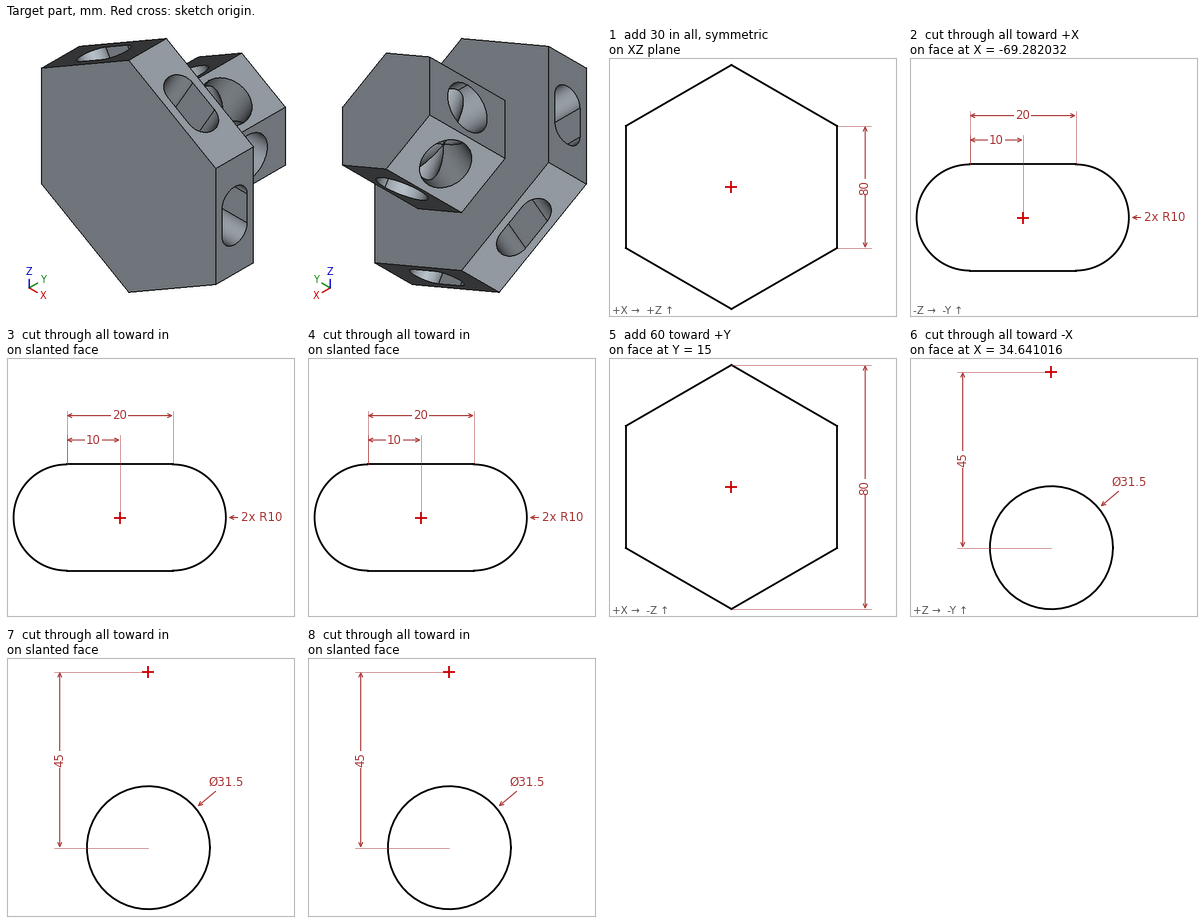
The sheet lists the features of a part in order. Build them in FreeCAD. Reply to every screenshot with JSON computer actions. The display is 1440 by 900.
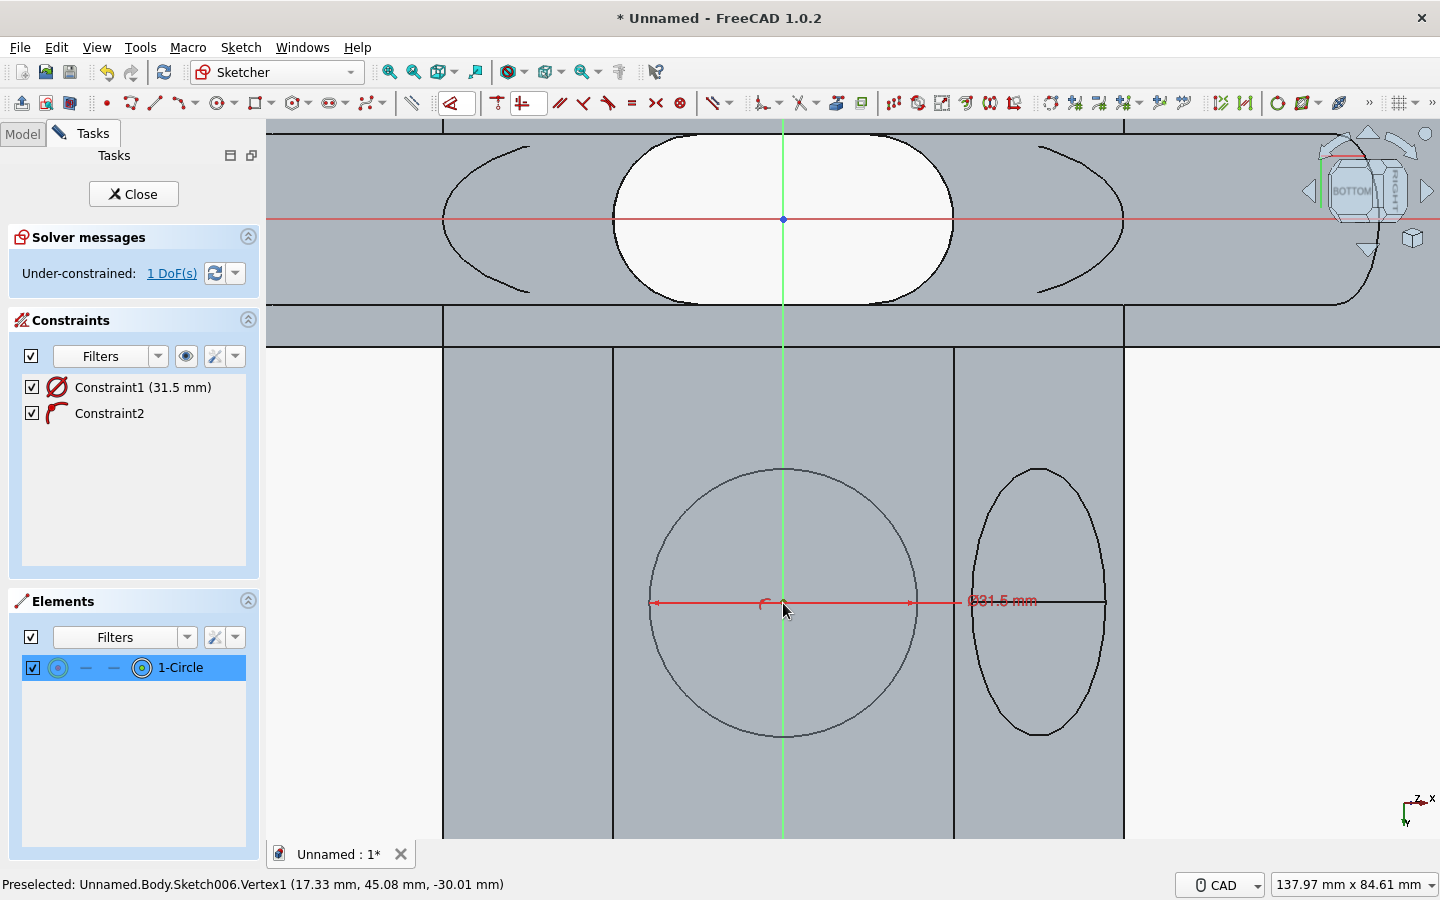
{"action": "left_click", "coordinate": [470, 104]}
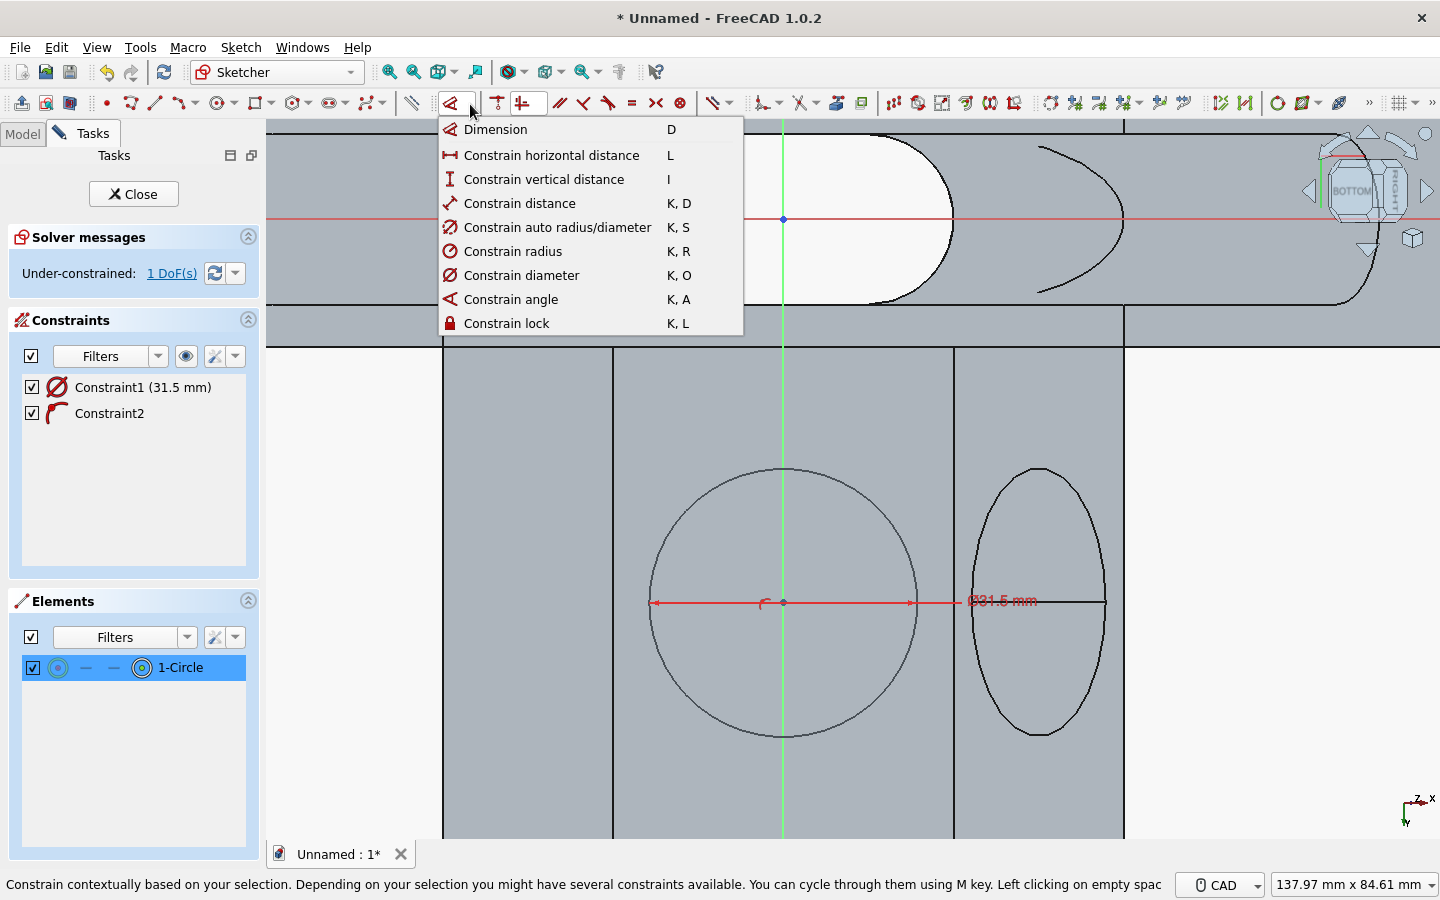
{"action": "left_click", "coordinate": [591, 179]}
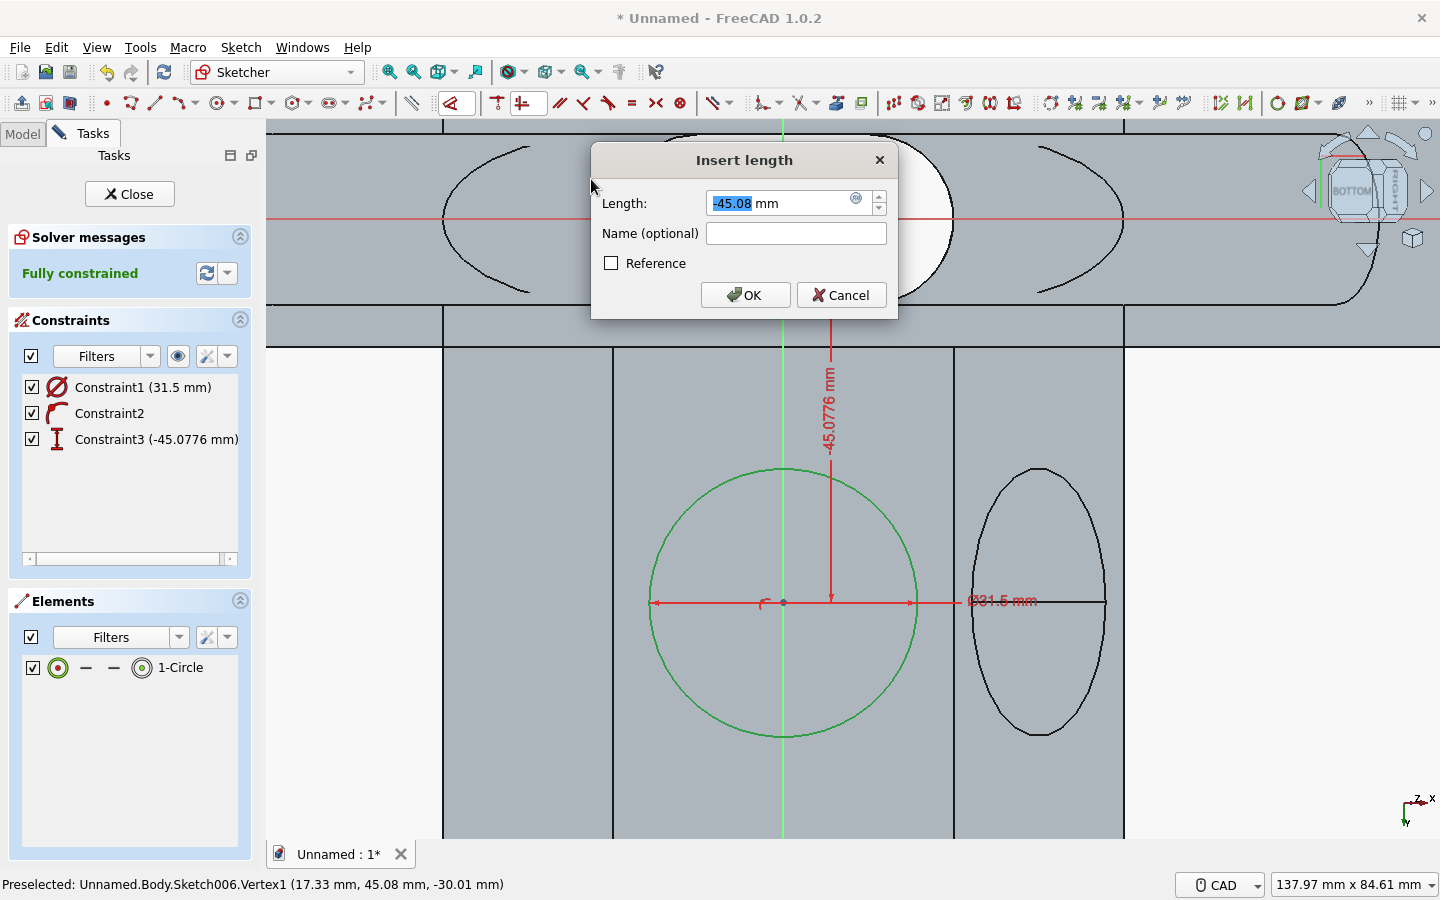
{"action": "type", "text": "-45"}
{"action": "key", "text": "Return"}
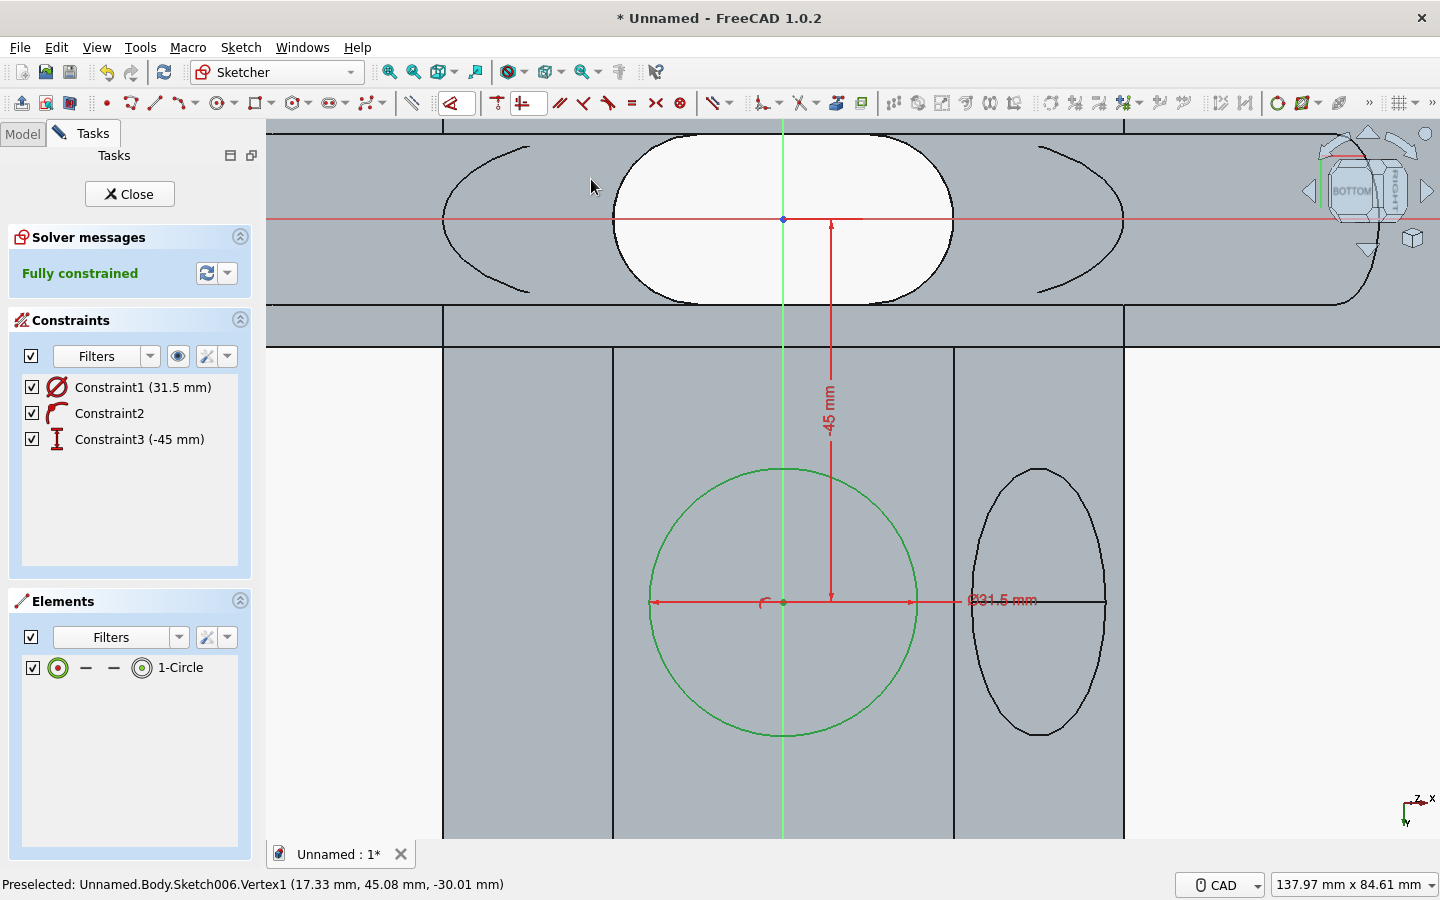
{"action": "left_click", "coordinate": [130, 194]}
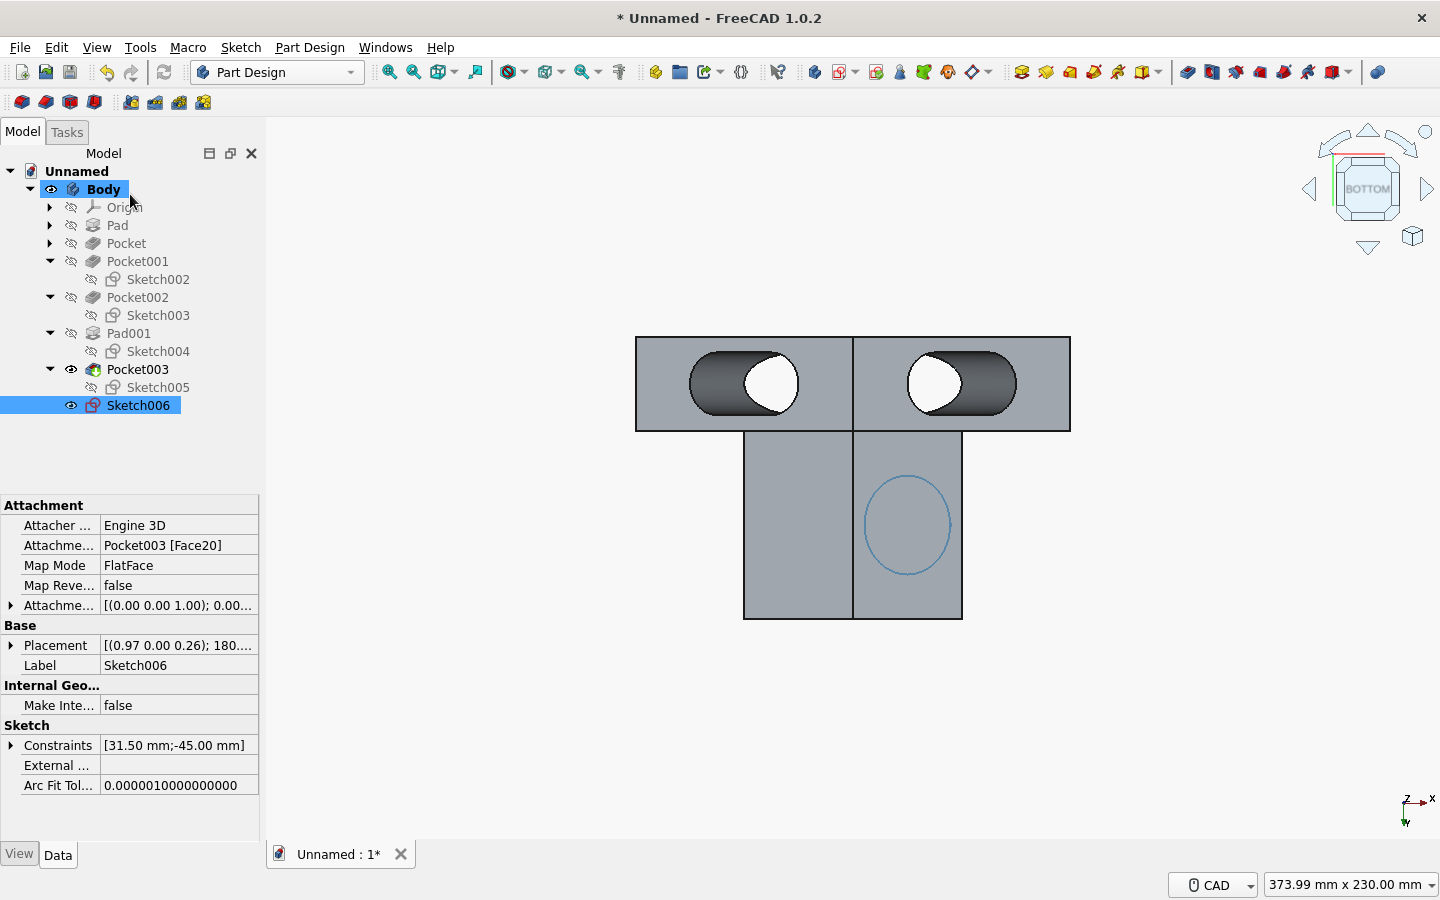
{"action": "left_click", "coordinate": [1188, 72]}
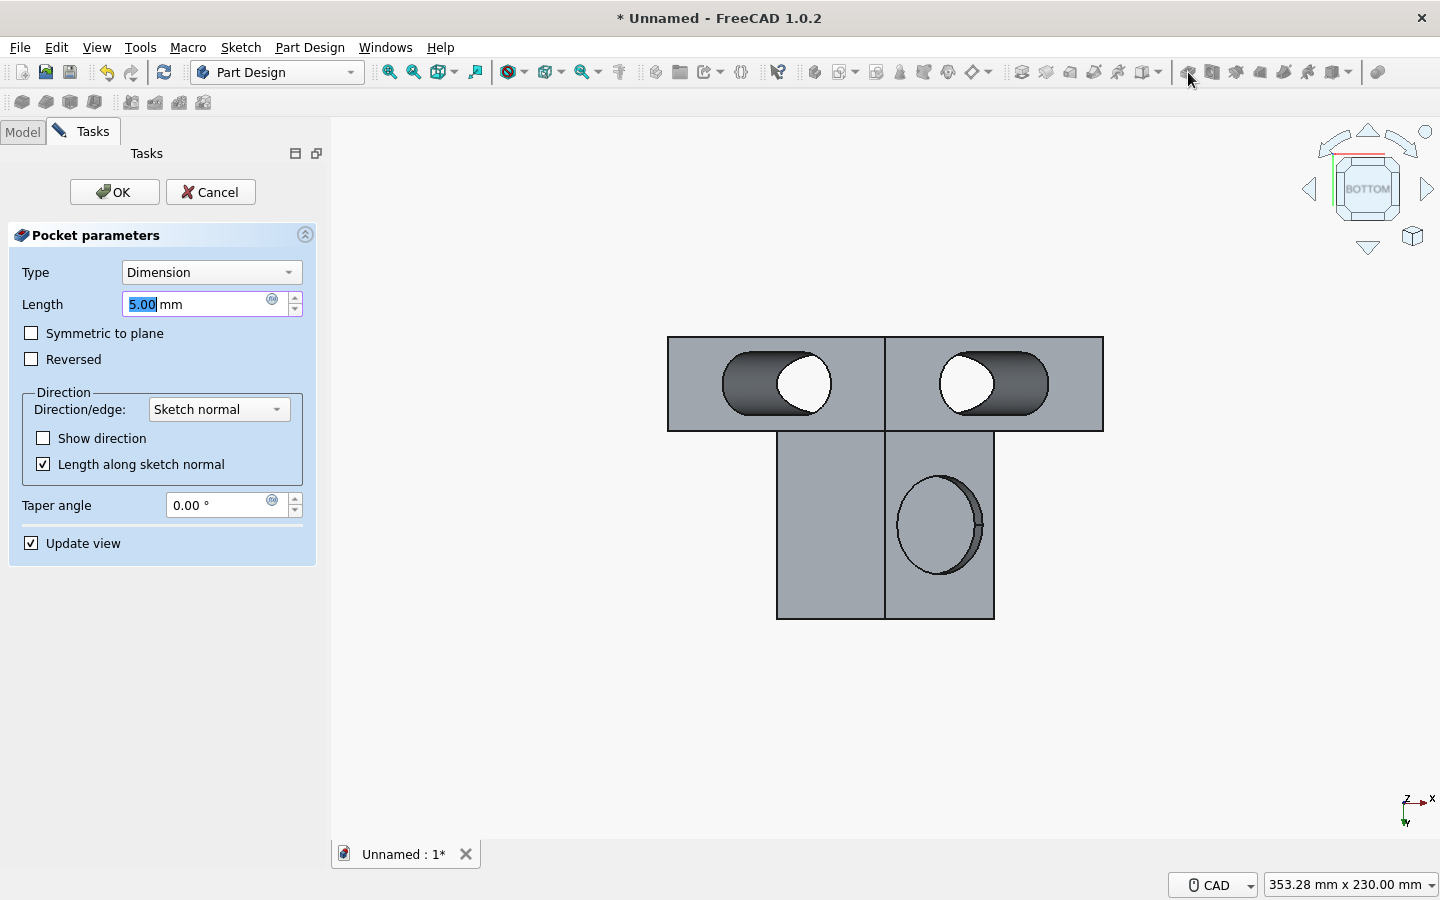
{"action": "left_click", "coordinate": [212, 272]}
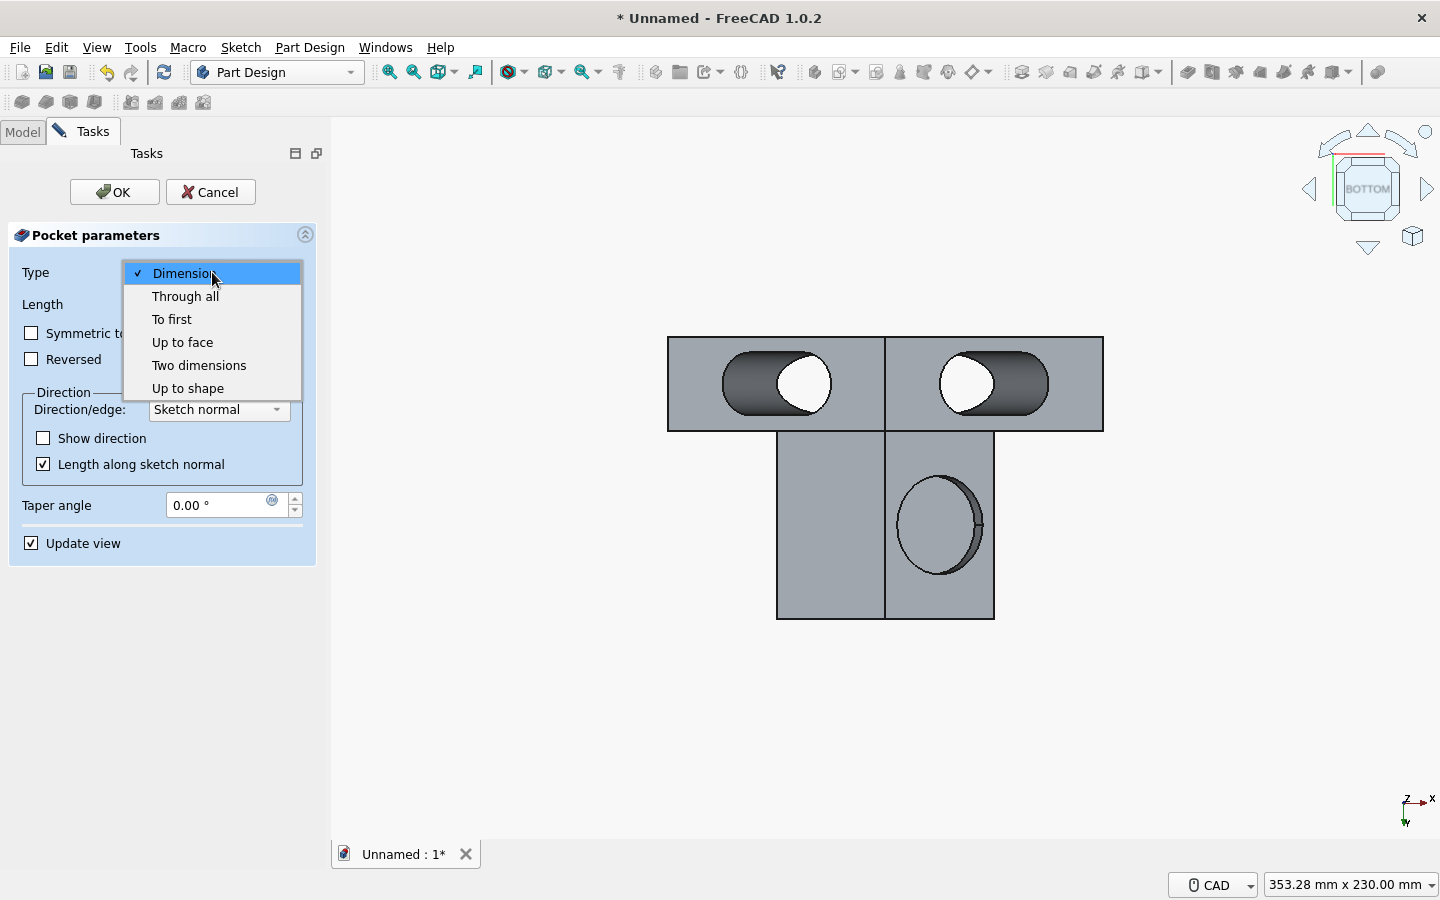
{"action": "left_click", "coordinate": [212, 296]}